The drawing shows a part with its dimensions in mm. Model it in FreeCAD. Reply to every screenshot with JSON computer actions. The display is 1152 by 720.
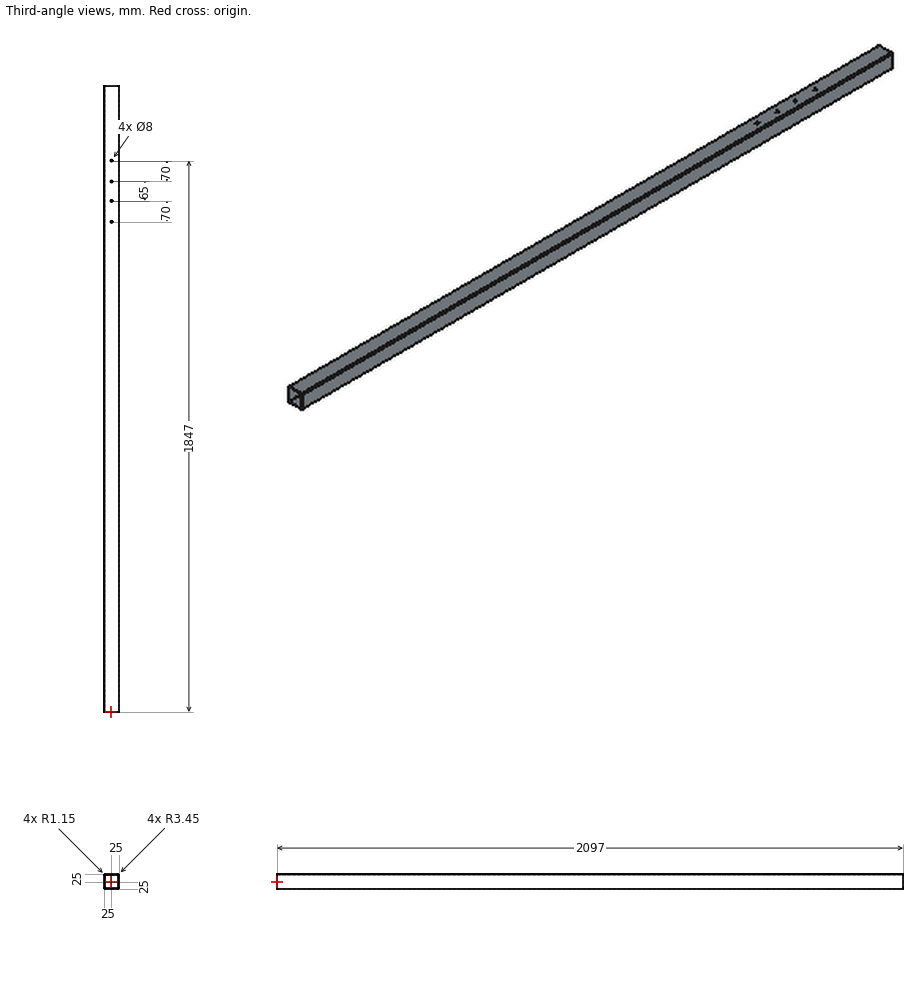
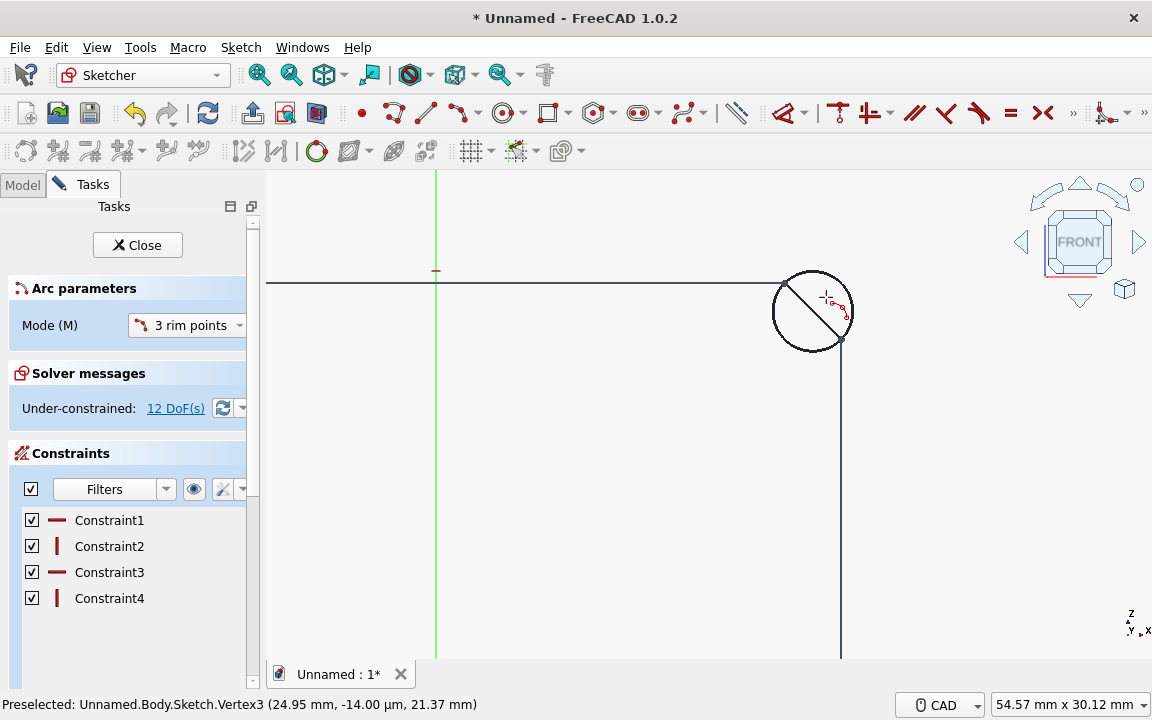
{"action": "left_click", "coordinate": [826, 297]}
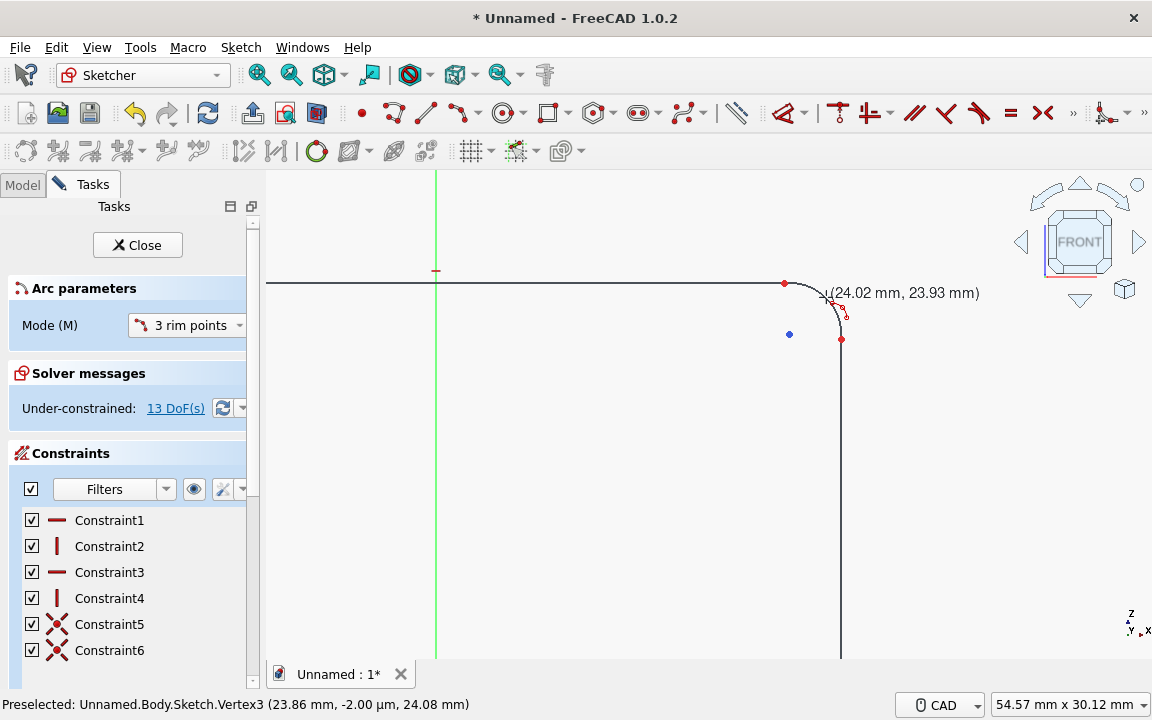
{"action": "scroll", "coordinate": [759, 256], "scroll_direction": "down", "scroll_amount": 5}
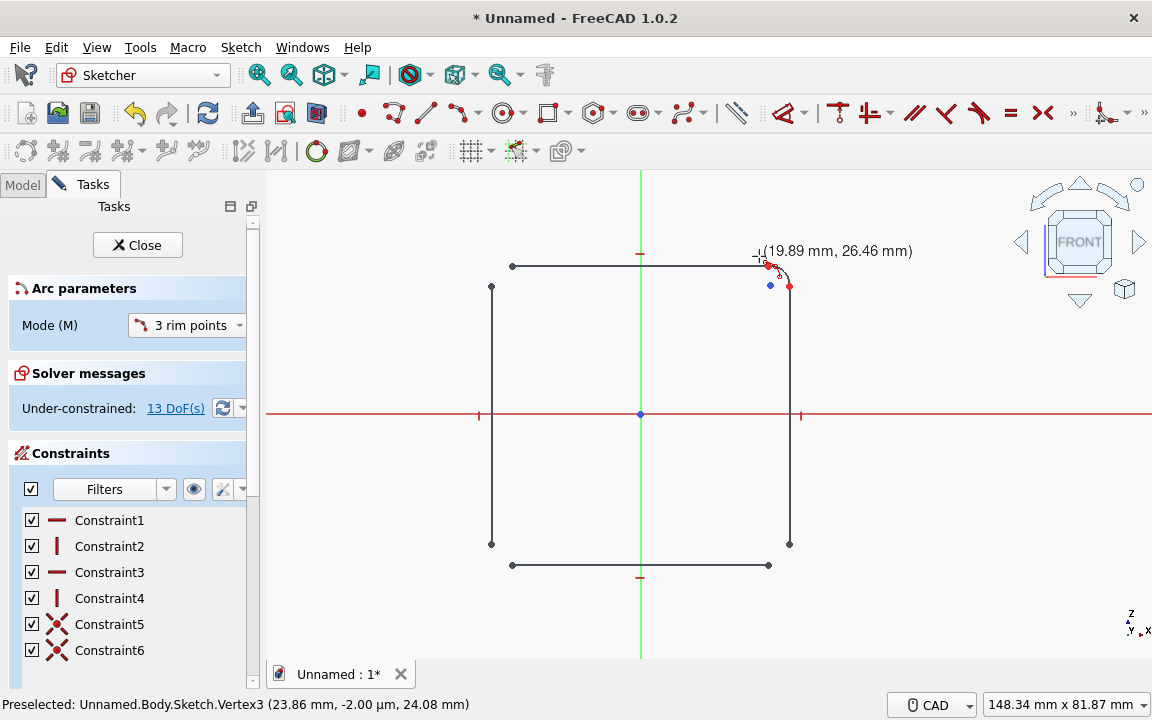
{"action": "left_click", "coordinate": [790, 545]}
{"action": "left_click", "coordinate": [769, 565]}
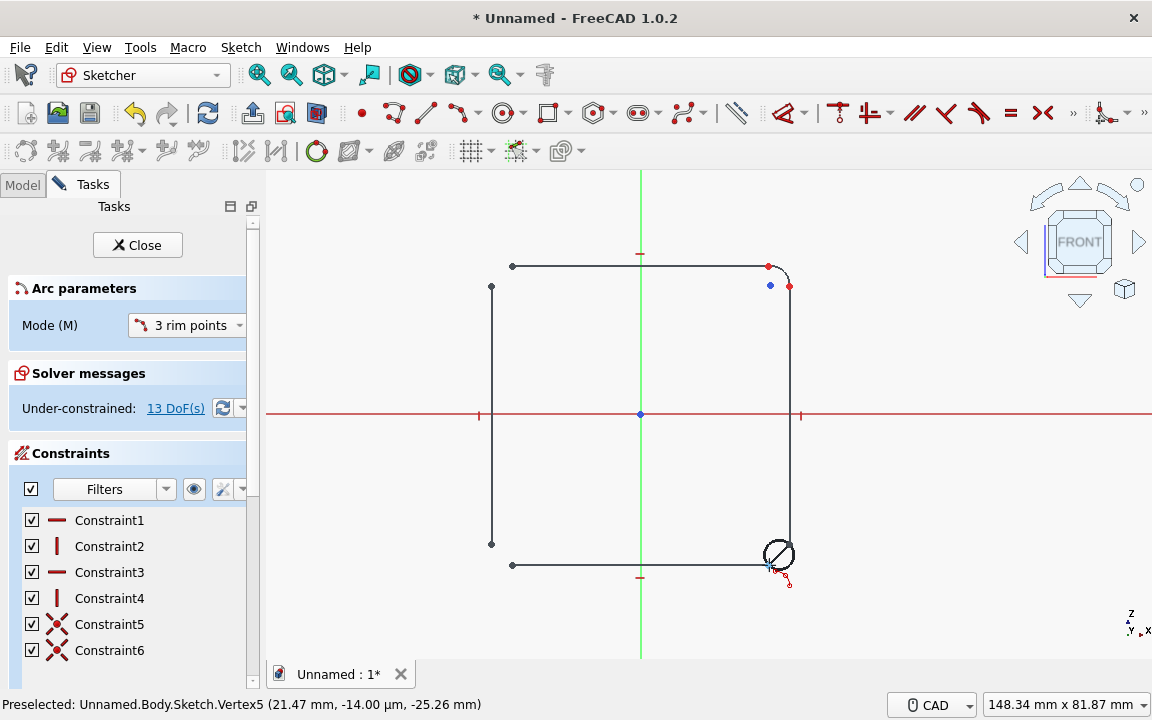
{"action": "scroll", "coordinate": [784, 558], "scroll_direction": "up", "scroll_amount": 5}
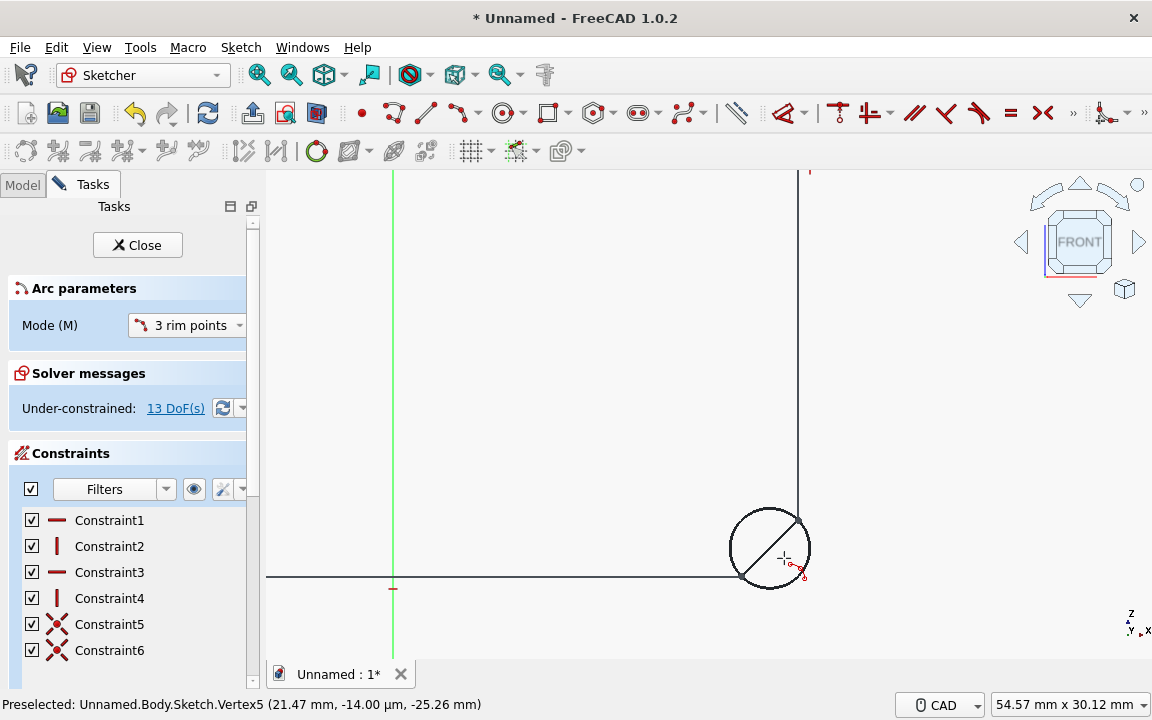
{"action": "left_click", "coordinate": [783, 556]}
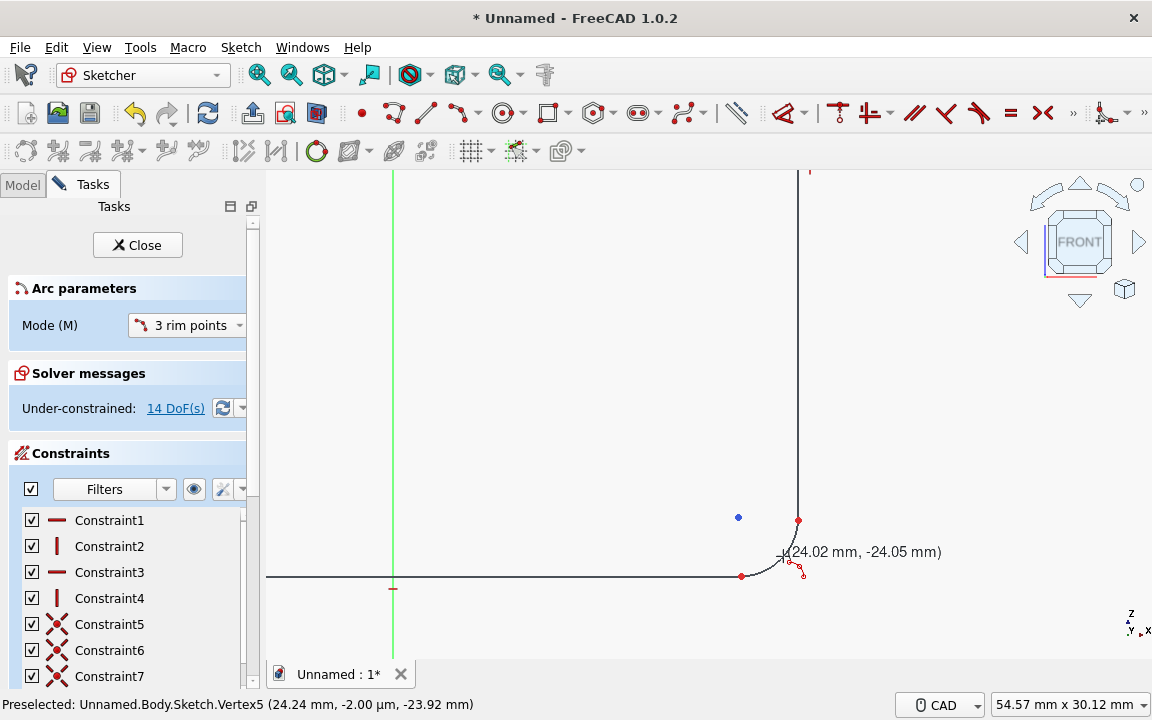
{"action": "scroll", "coordinate": [784, 559], "scroll_direction": "down", "scroll_amount": 5}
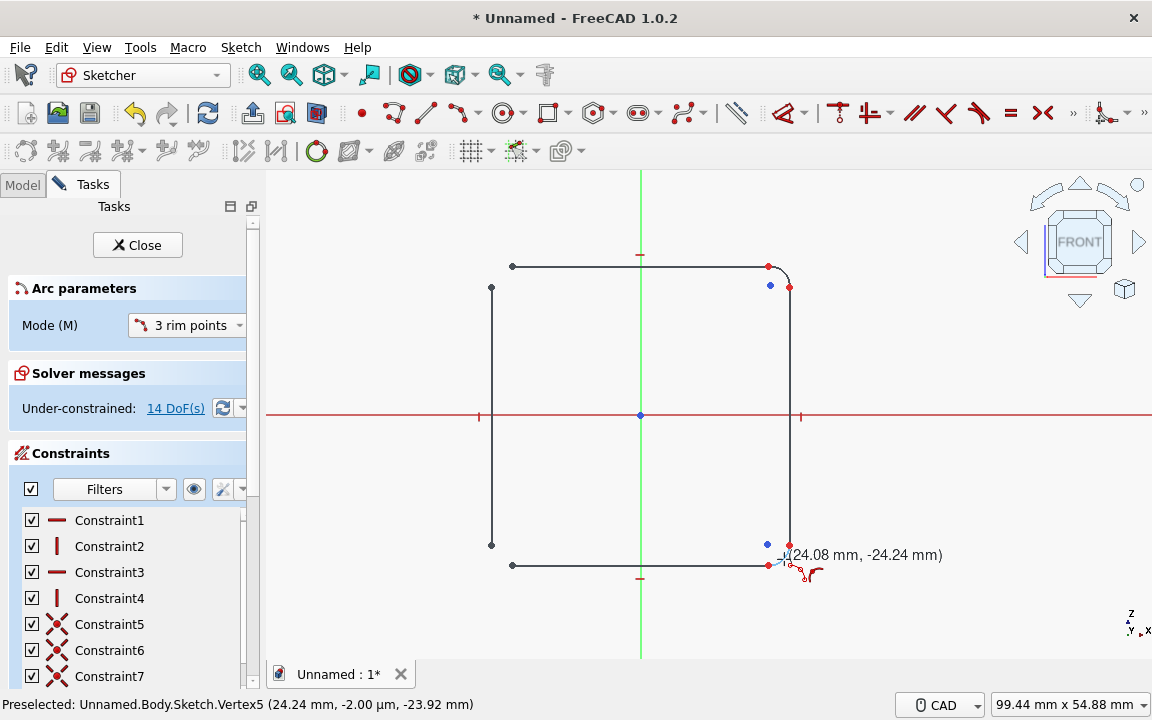
{"action": "left_click", "coordinate": [512, 566]}
{"action": "left_click", "coordinate": [492, 545]}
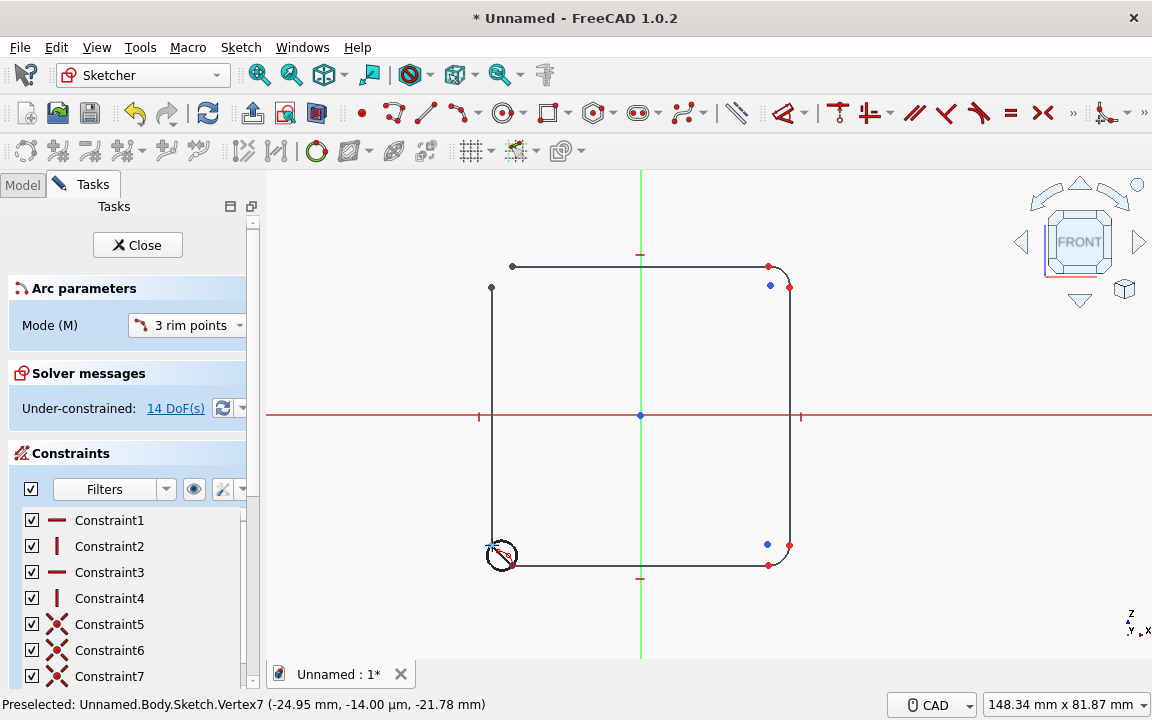
{"action": "scroll", "coordinate": [497, 558], "scroll_direction": "up", "scroll_amount": 5}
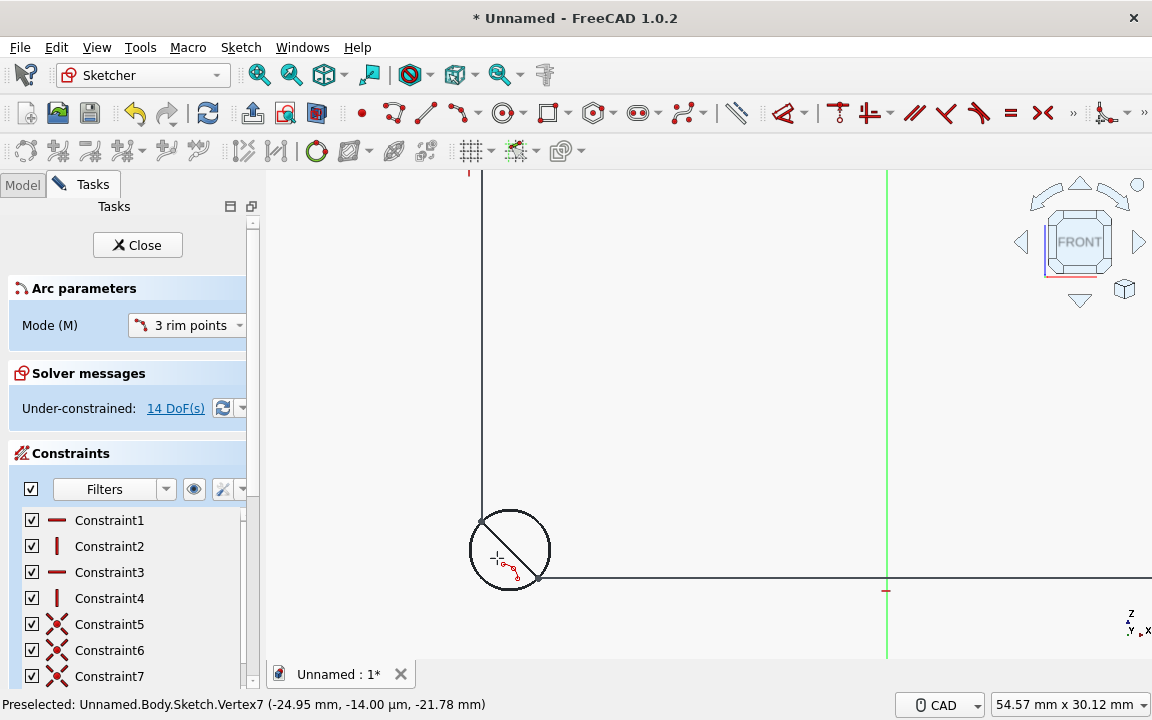
{"action": "left_click", "coordinate": [497, 558]}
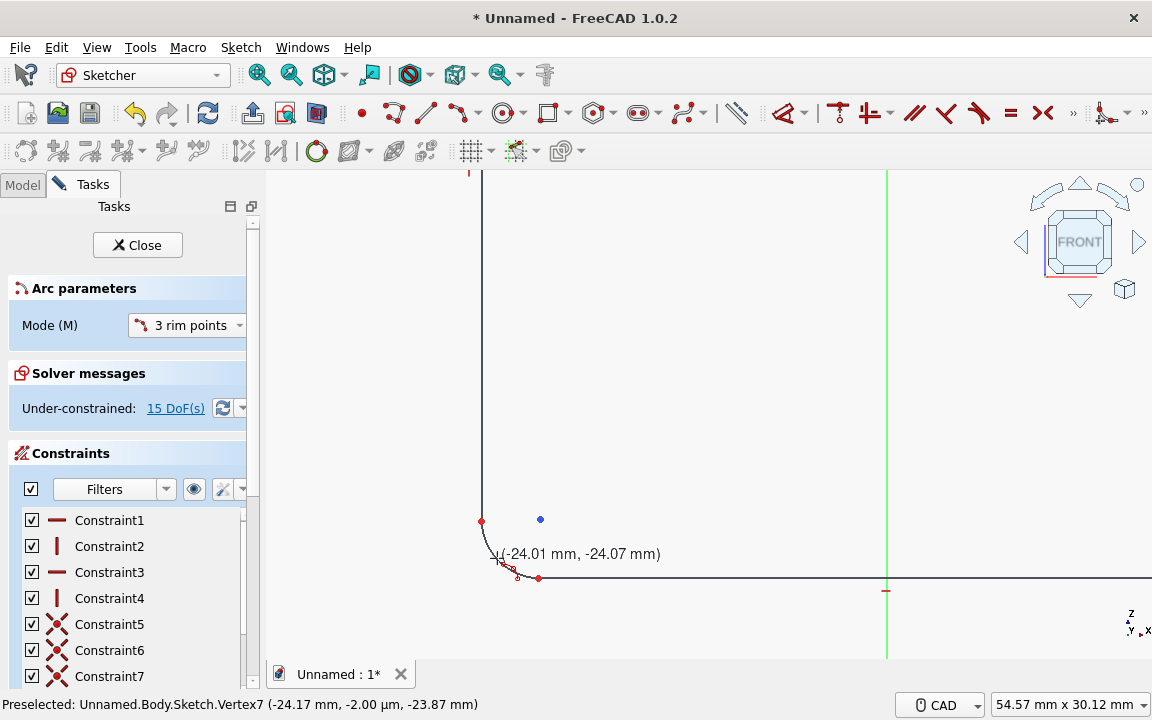
{"action": "scroll", "coordinate": [497, 558], "scroll_direction": "down", "scroll_amount": 5}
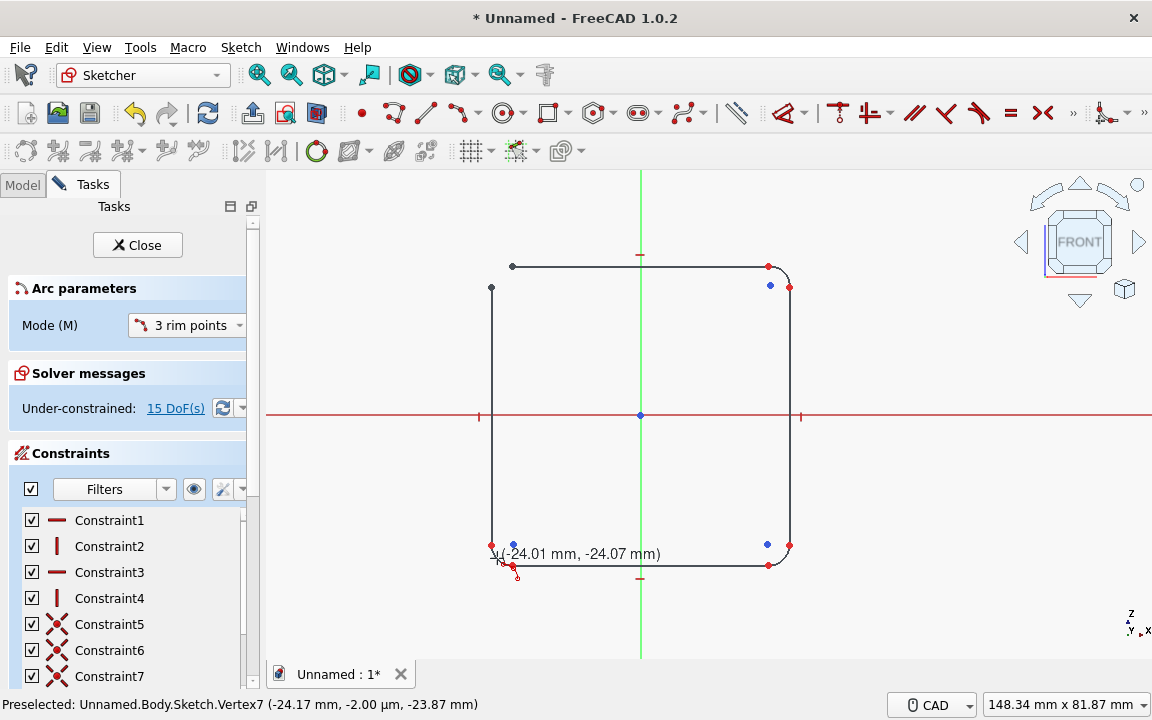
{"action": "left_click", "coordinate": [492, 287]}
{"action": "left_click", "coordinate": [512, 267]}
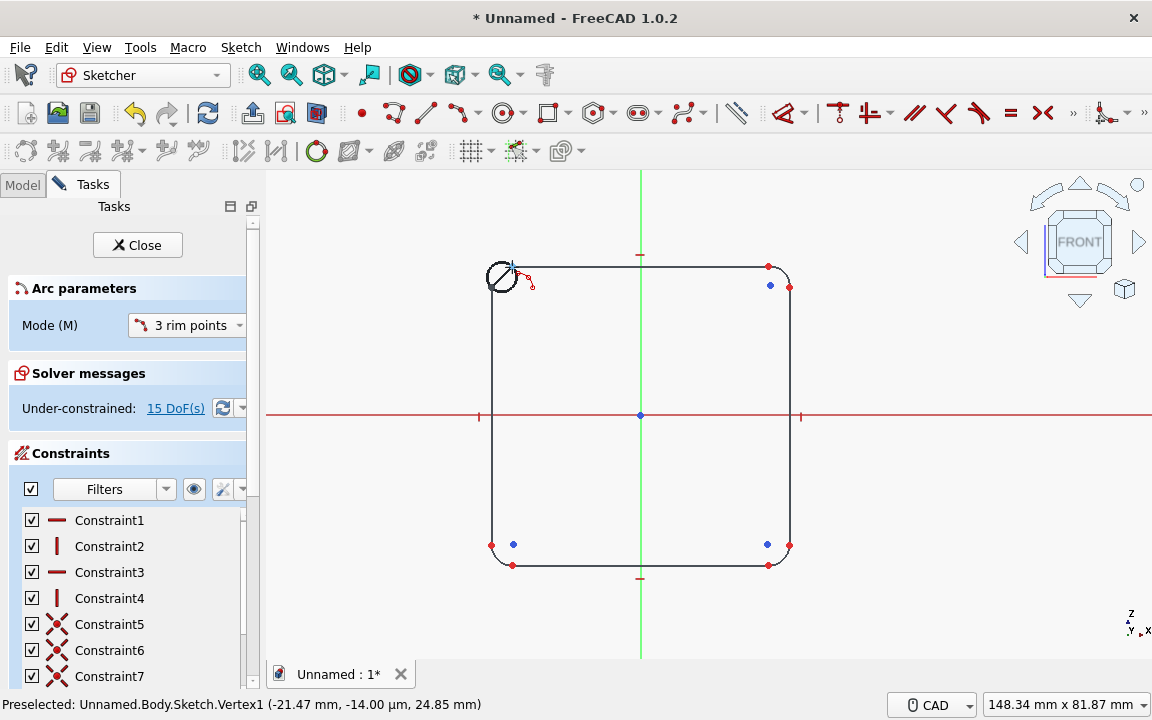
{"action": "scroll", "coordinate": [497, 272], "scroll_direction": "up", "scroll_amount": 5}